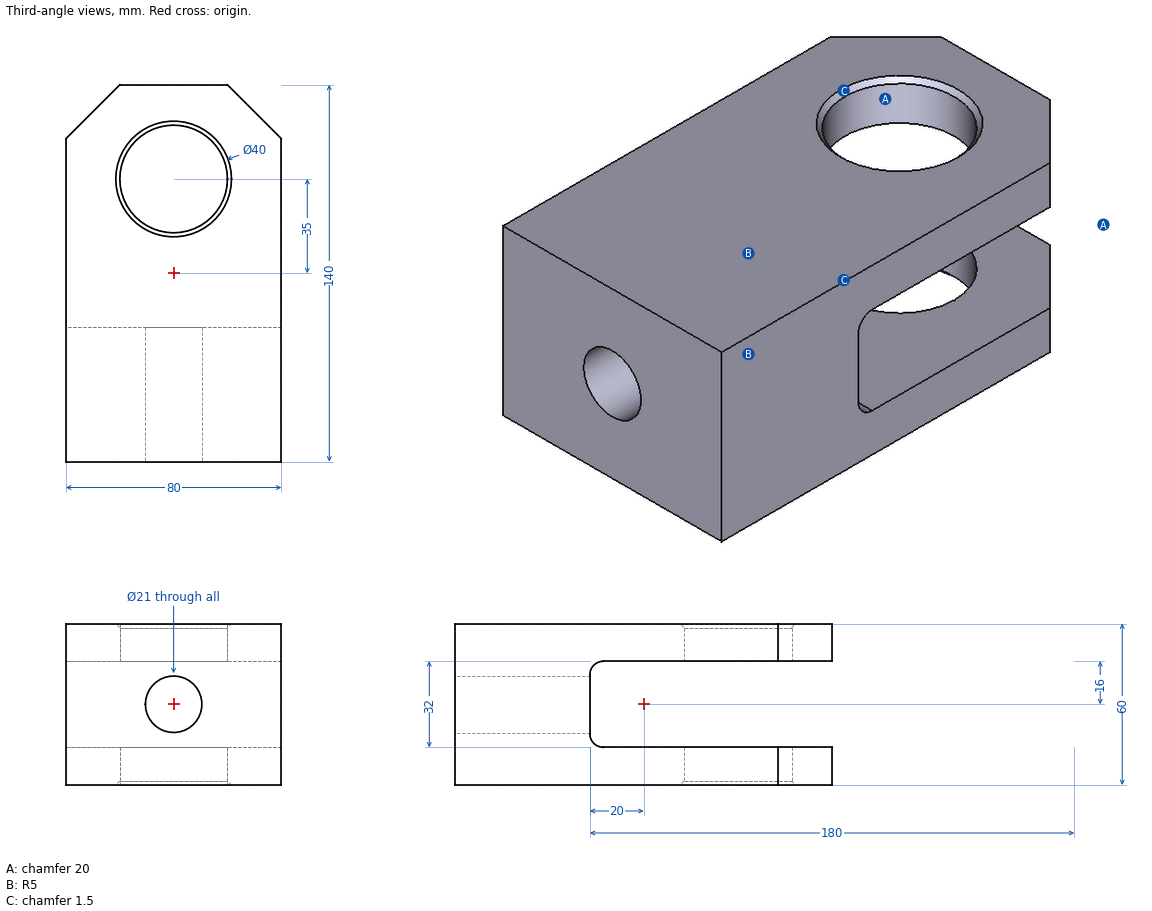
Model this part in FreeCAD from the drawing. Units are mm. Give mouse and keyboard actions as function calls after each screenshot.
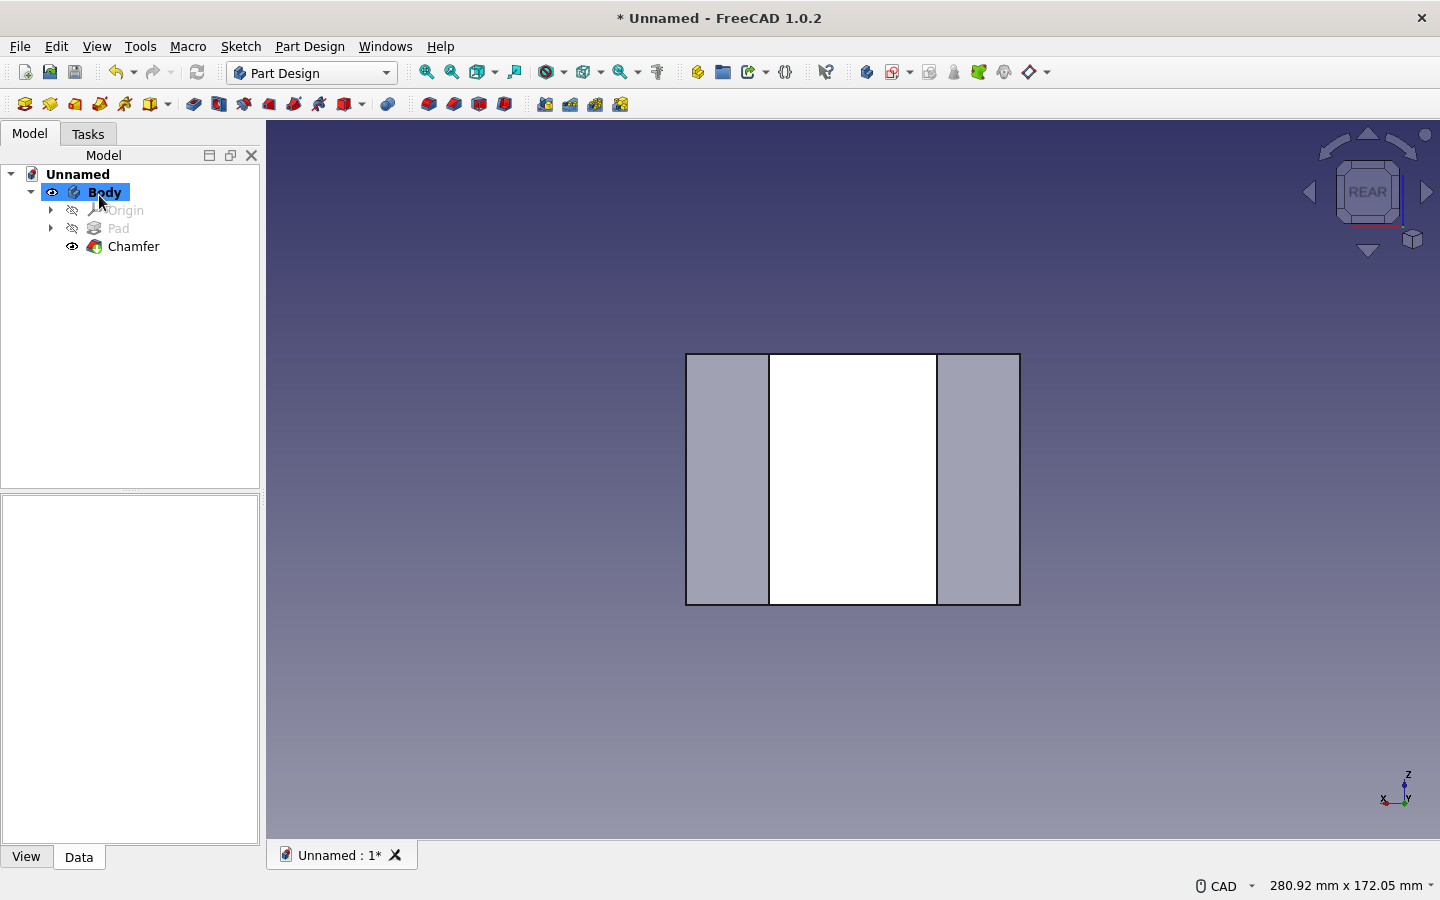
click(427, 72)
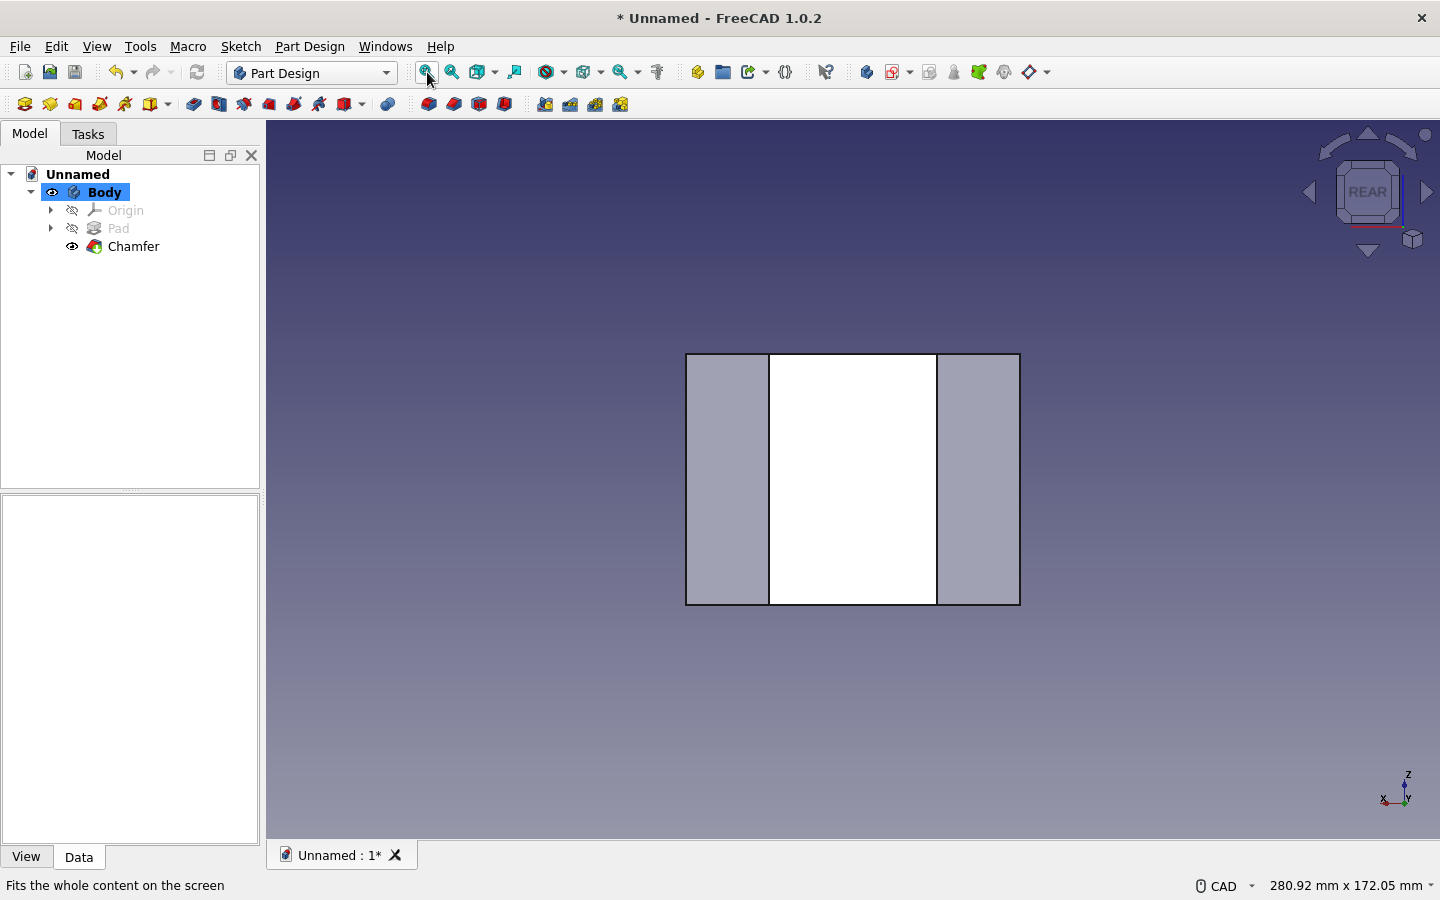
key(6)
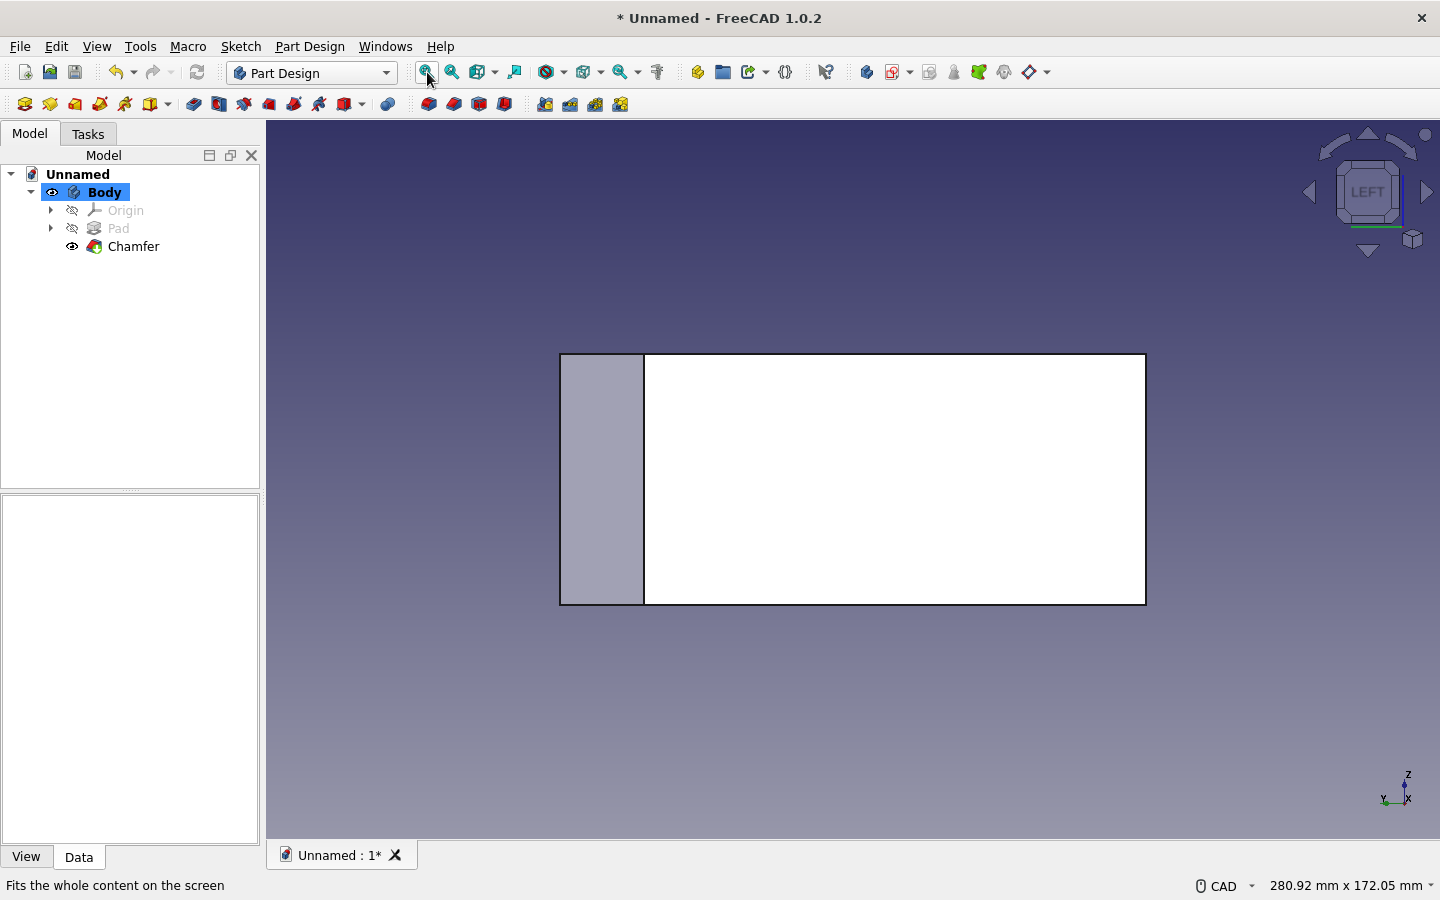
click(823, 478)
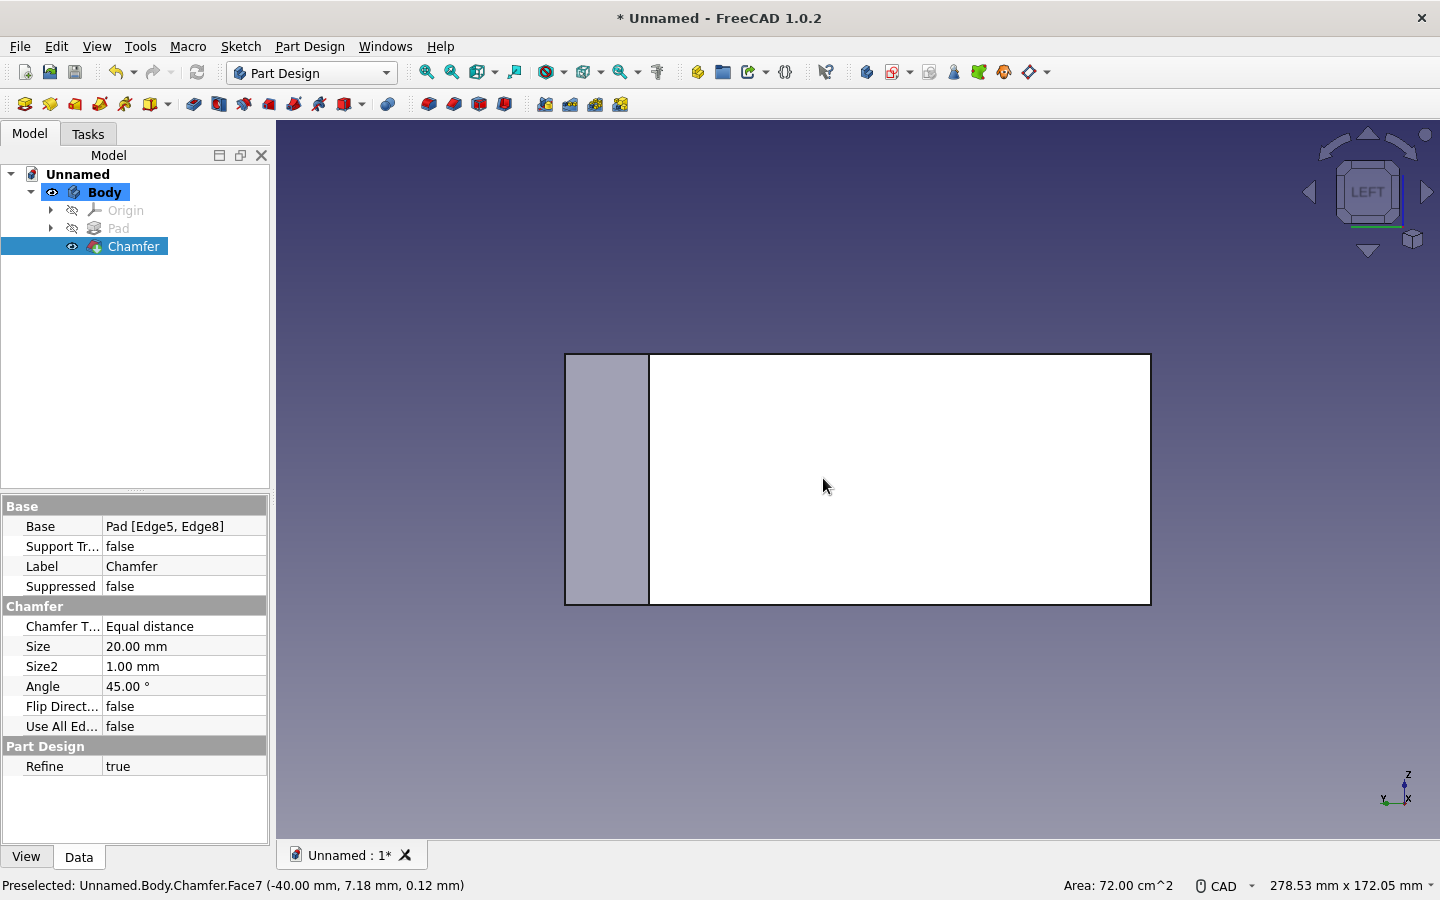
click(892, 72)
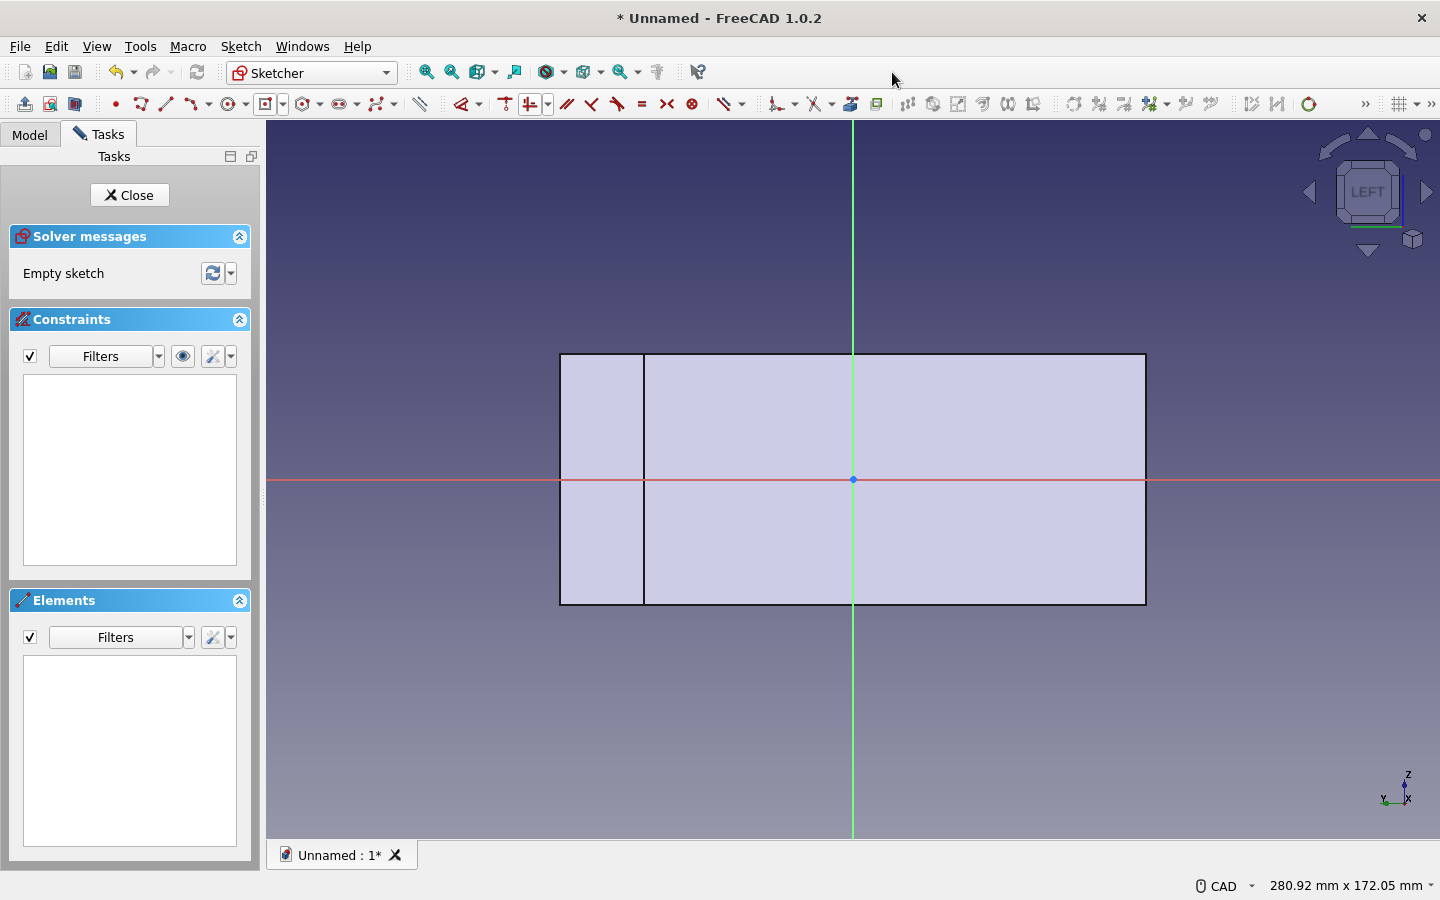
scroll(1275, 480, down, 1)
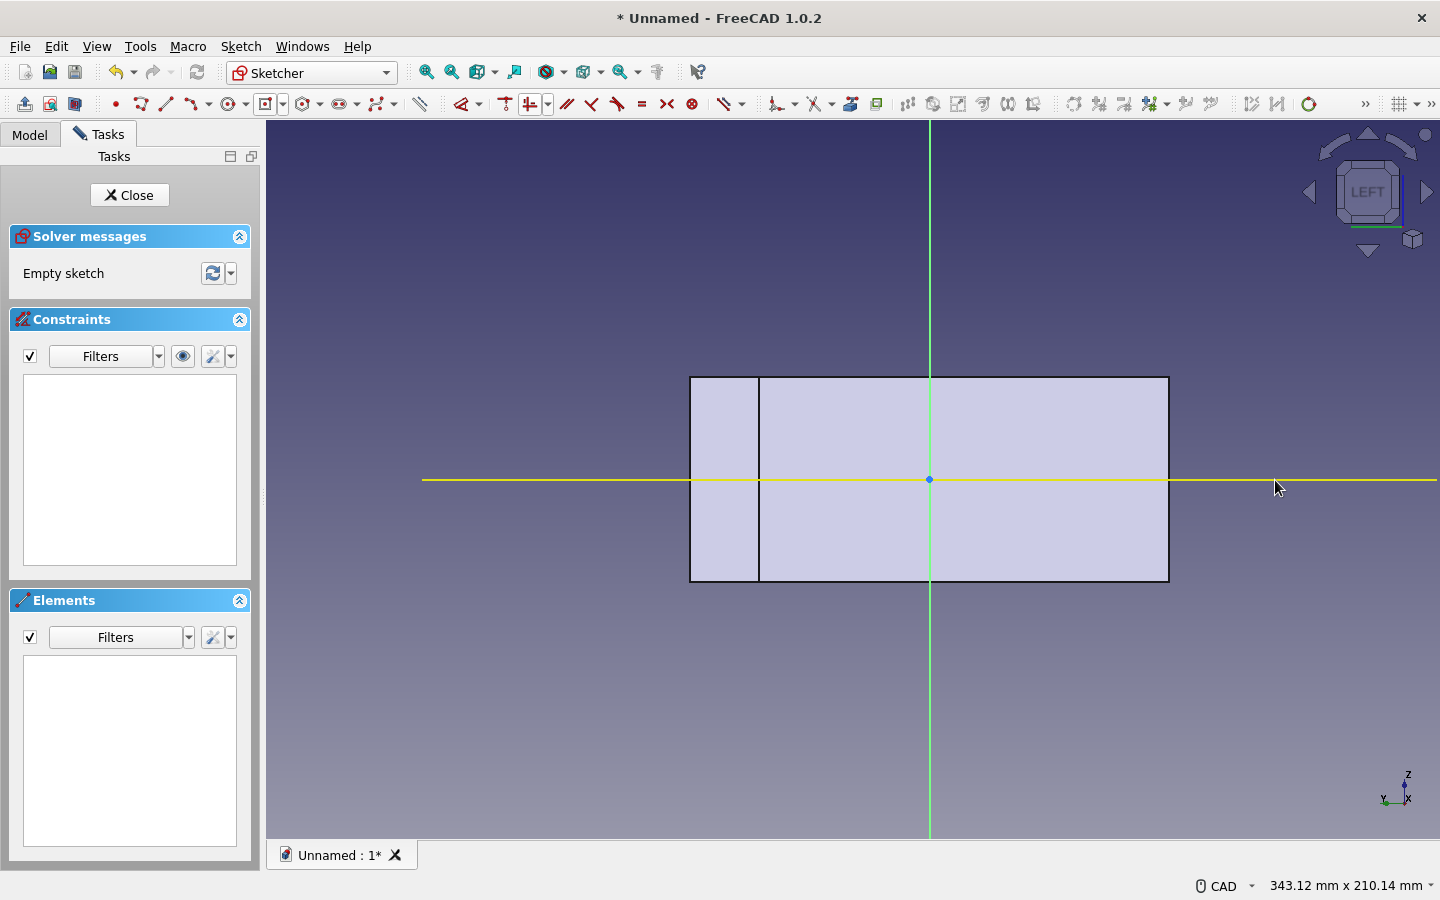
click(282, 104)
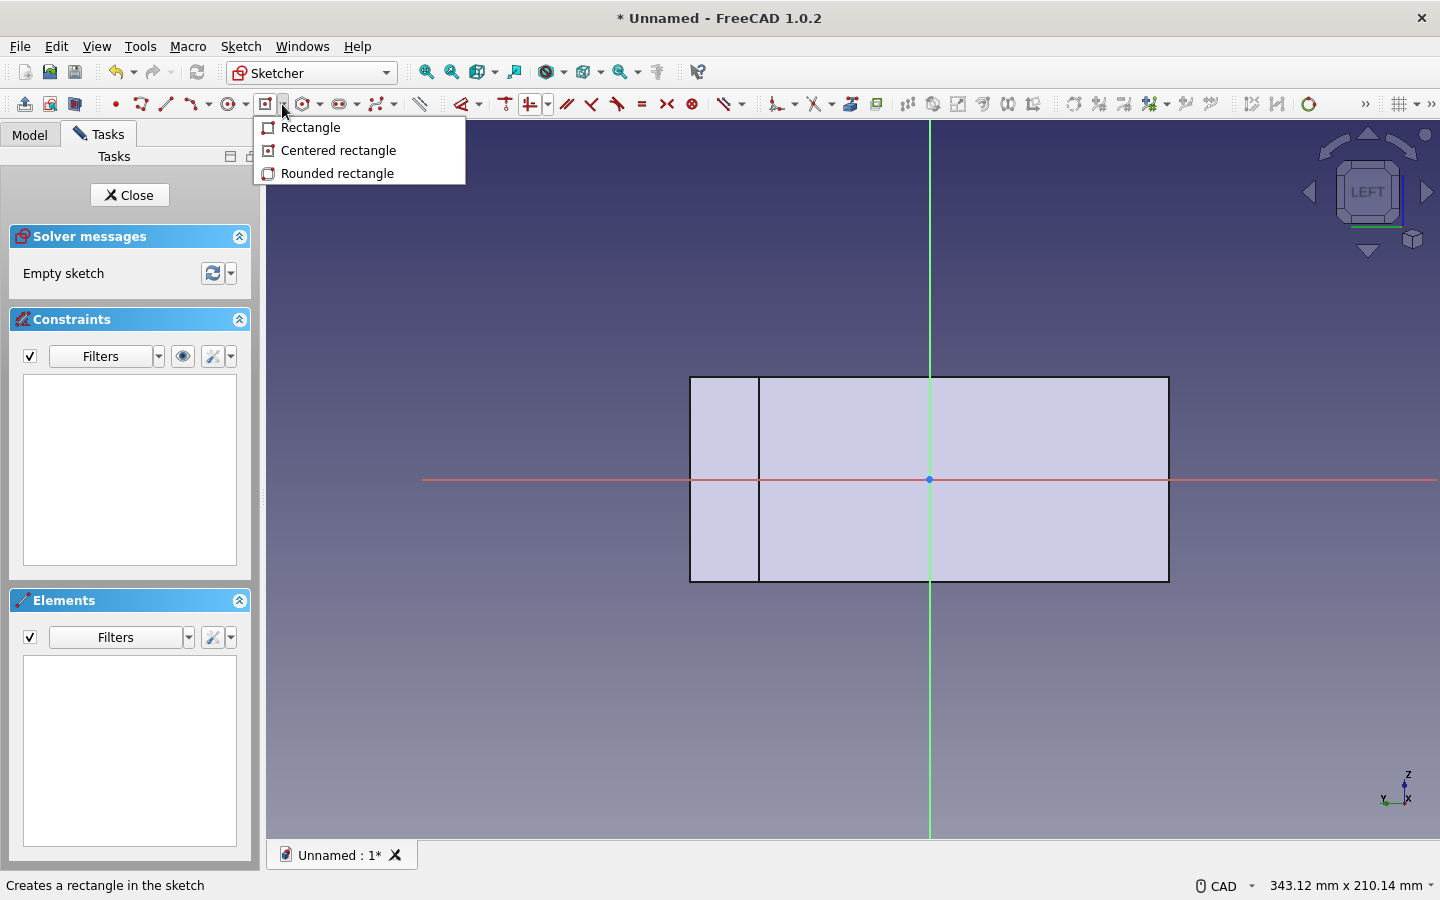
click(360, 128)